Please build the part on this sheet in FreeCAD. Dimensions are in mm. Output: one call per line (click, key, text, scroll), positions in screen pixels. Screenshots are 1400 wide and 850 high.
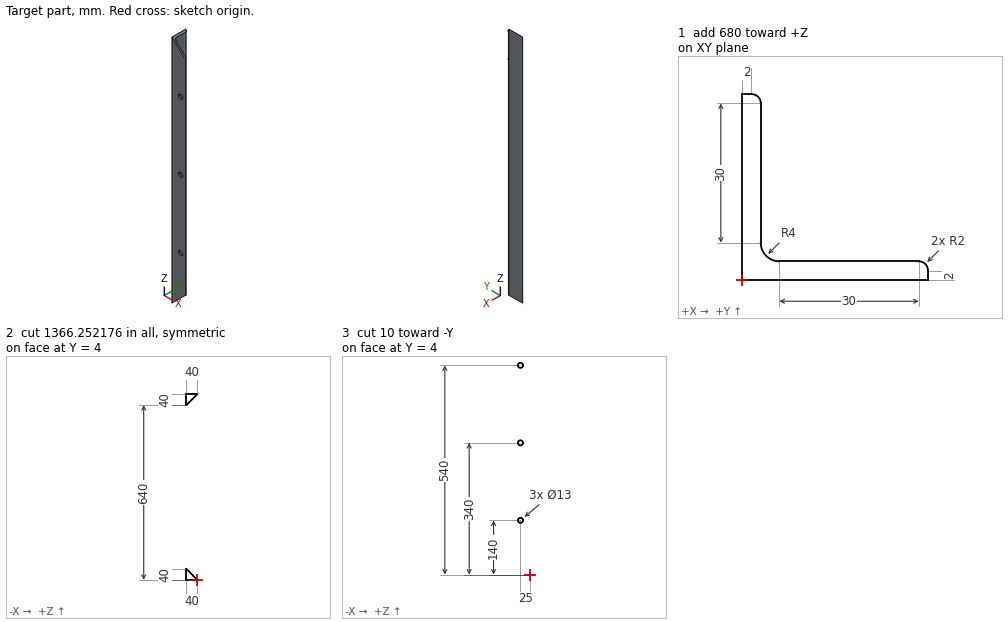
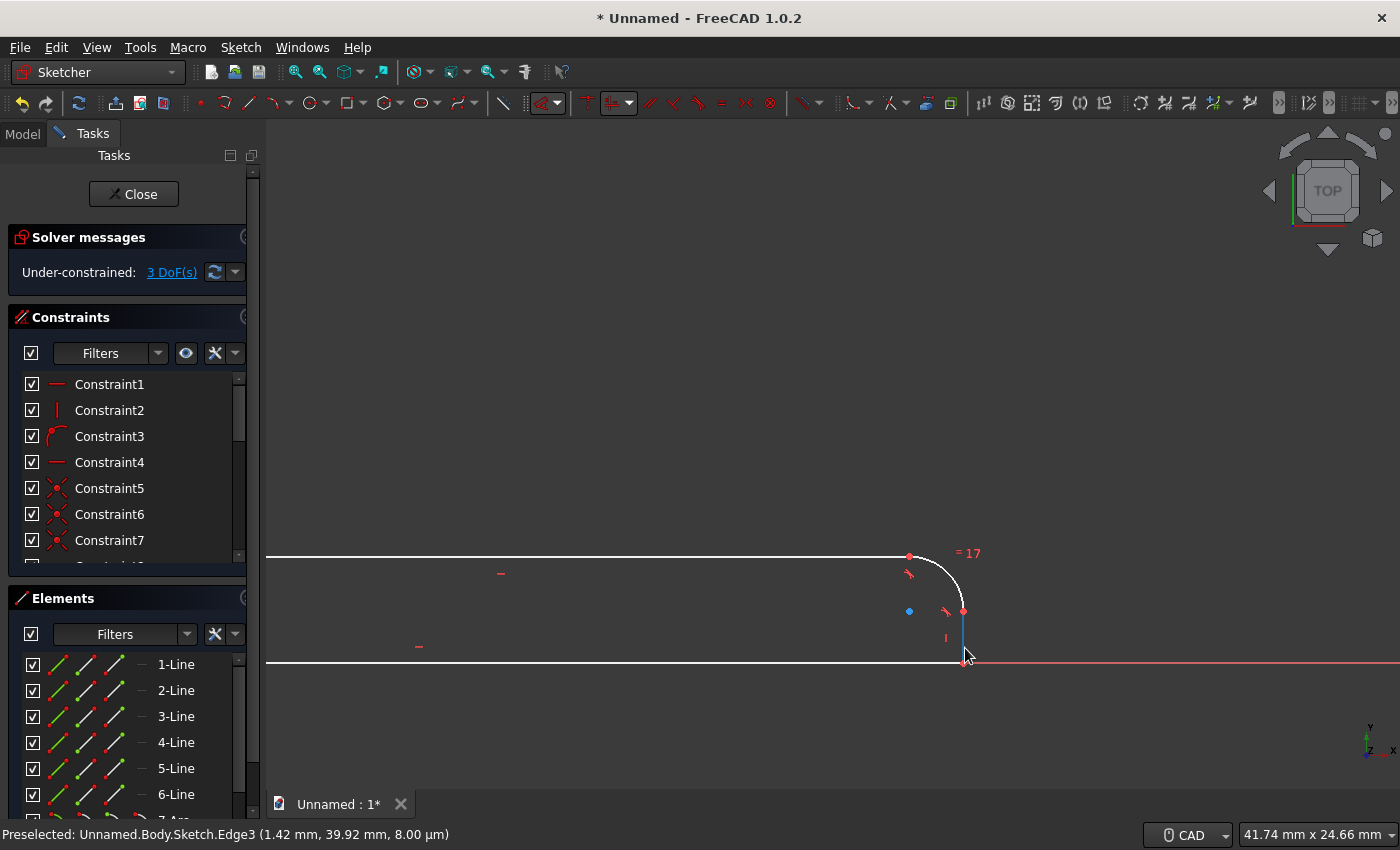
click(963, 648)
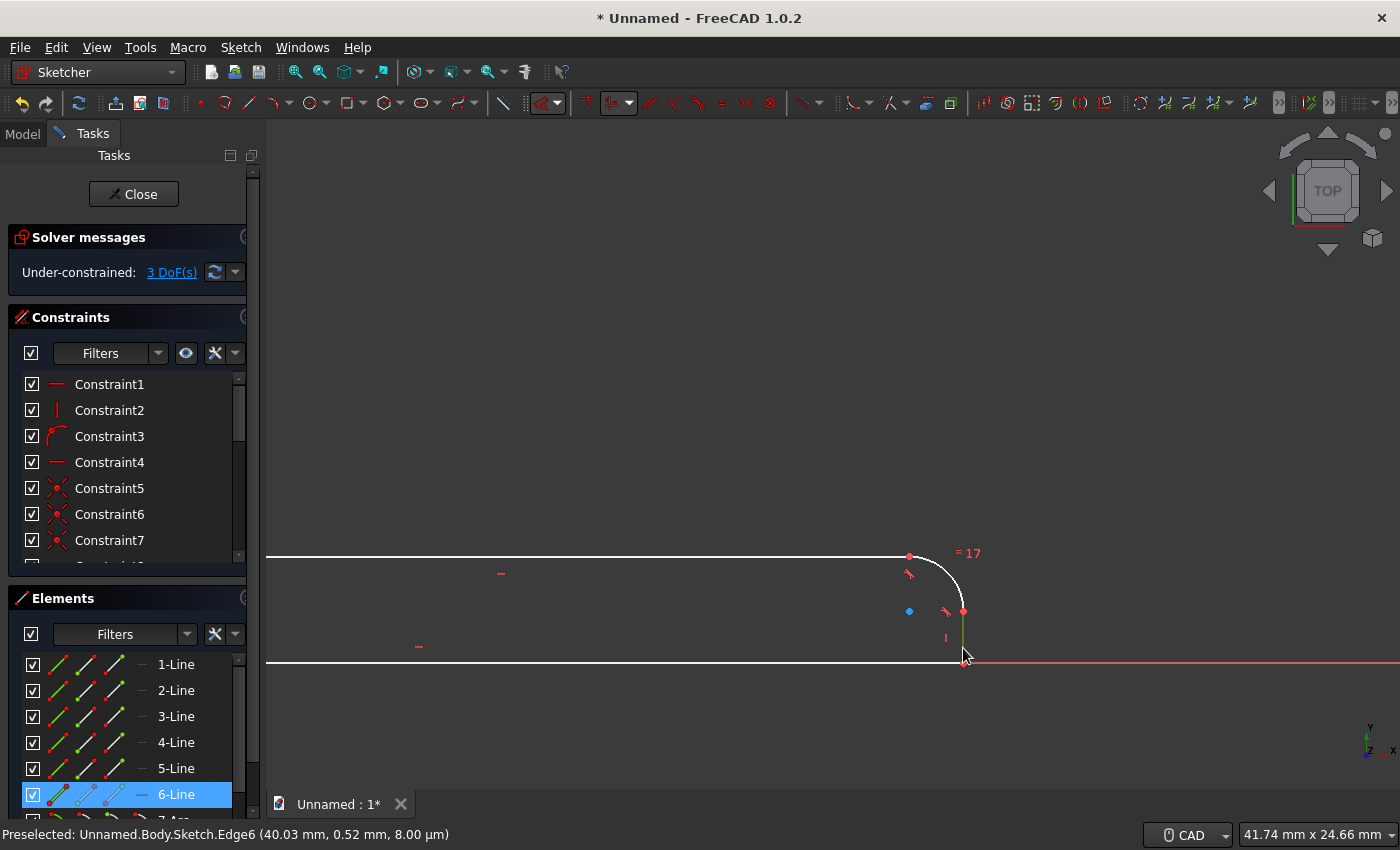
click(560, 104)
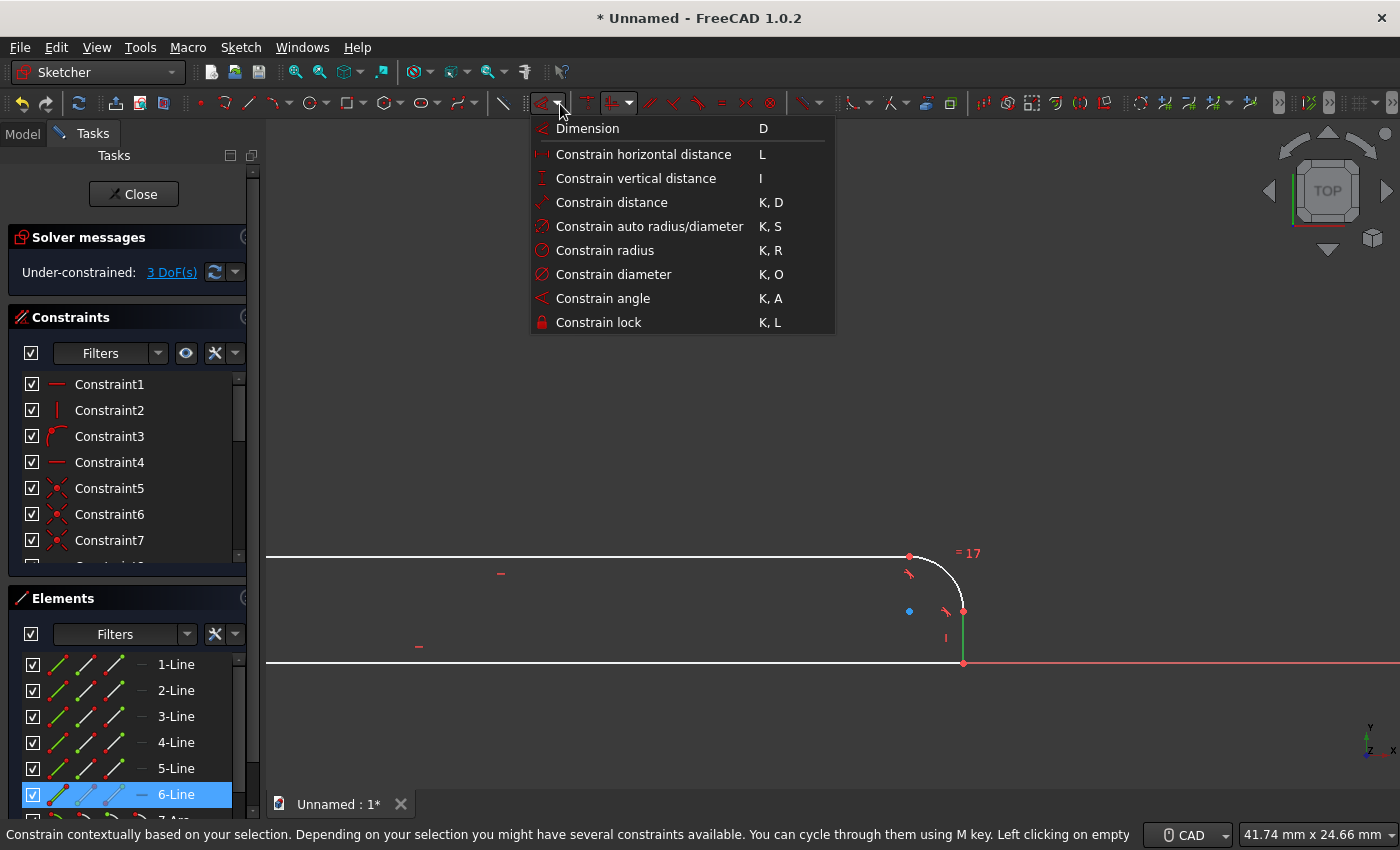
click(683, 178)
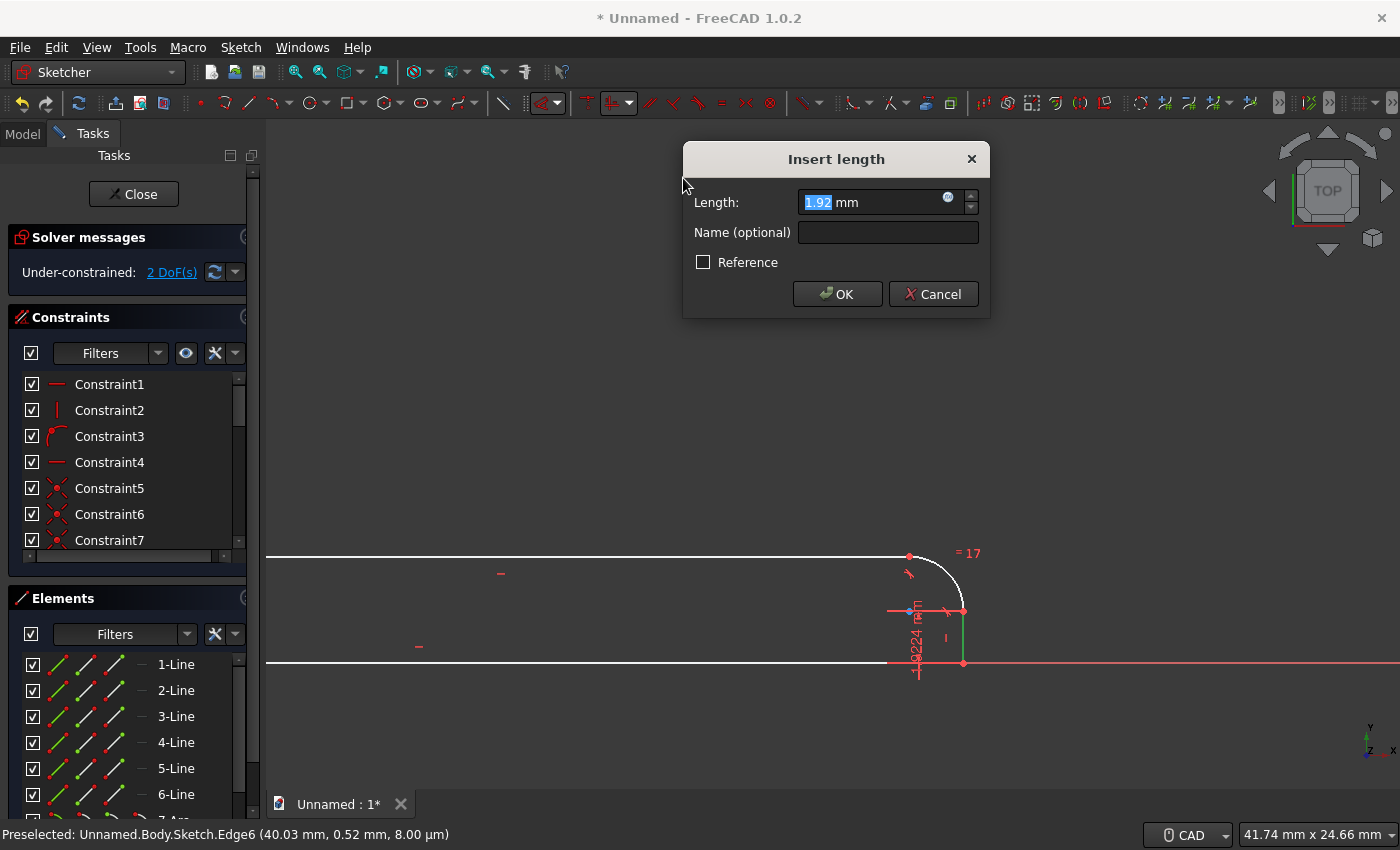
text(2)
key(Return)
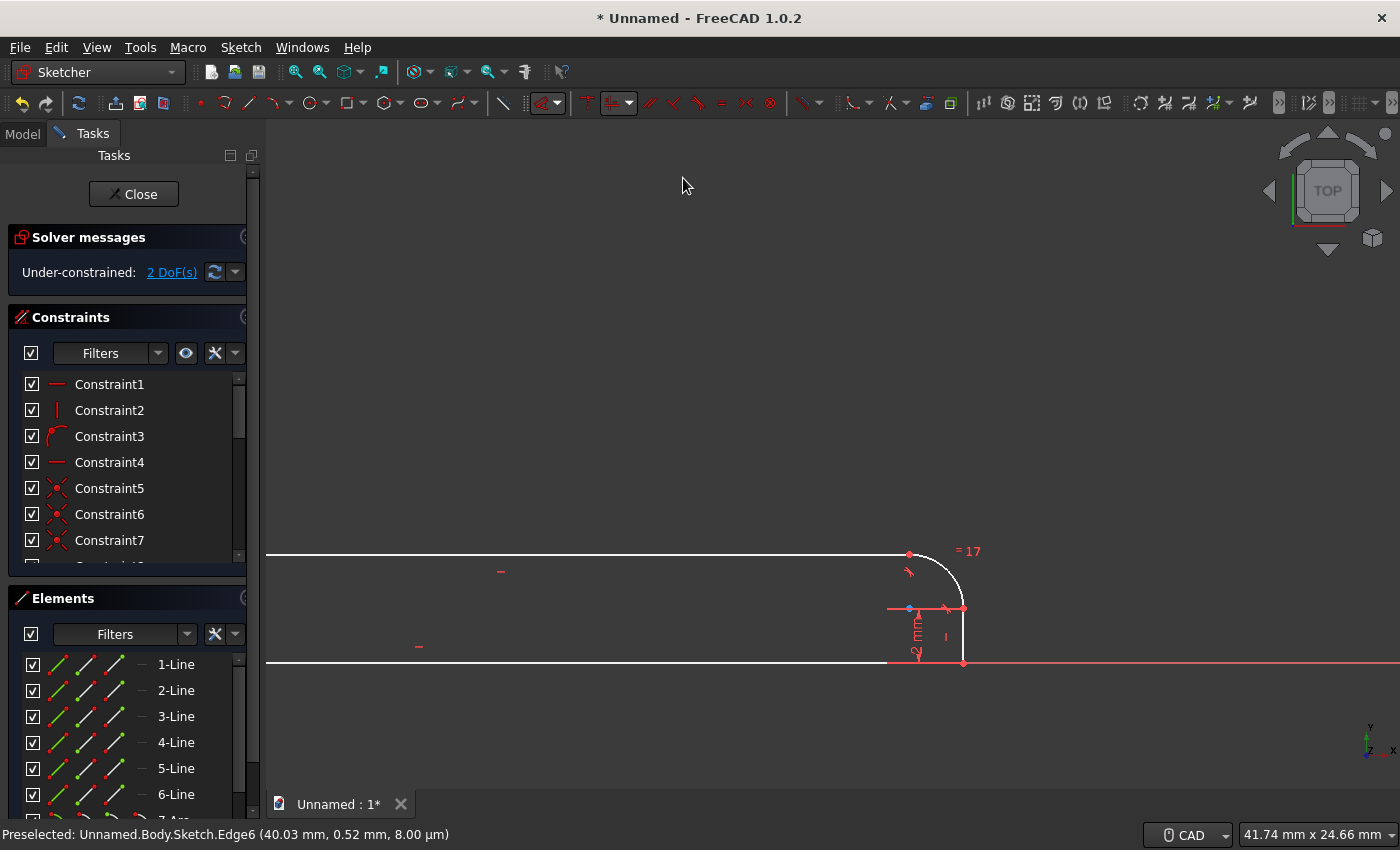
click(664, 555)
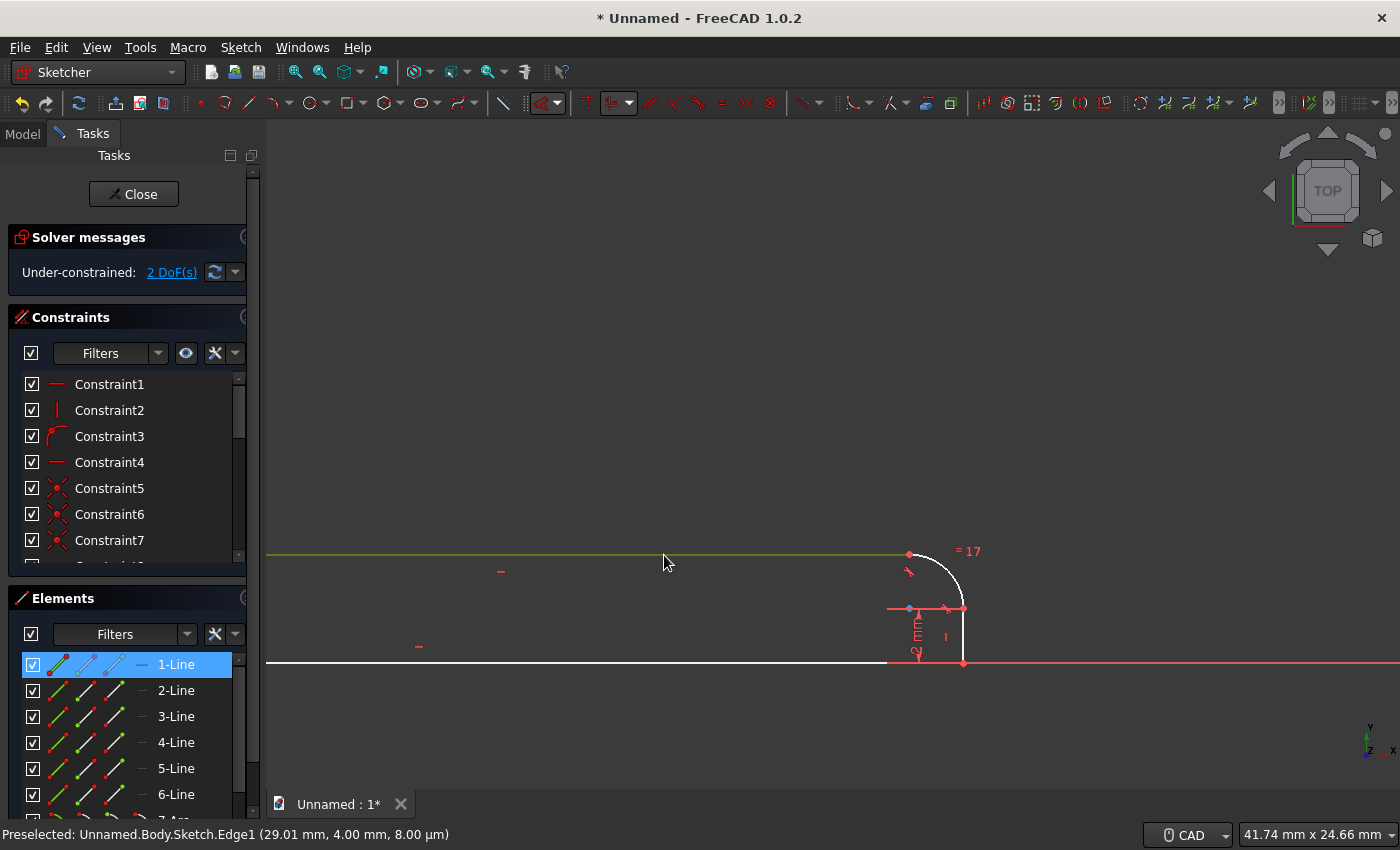
click(560, 104)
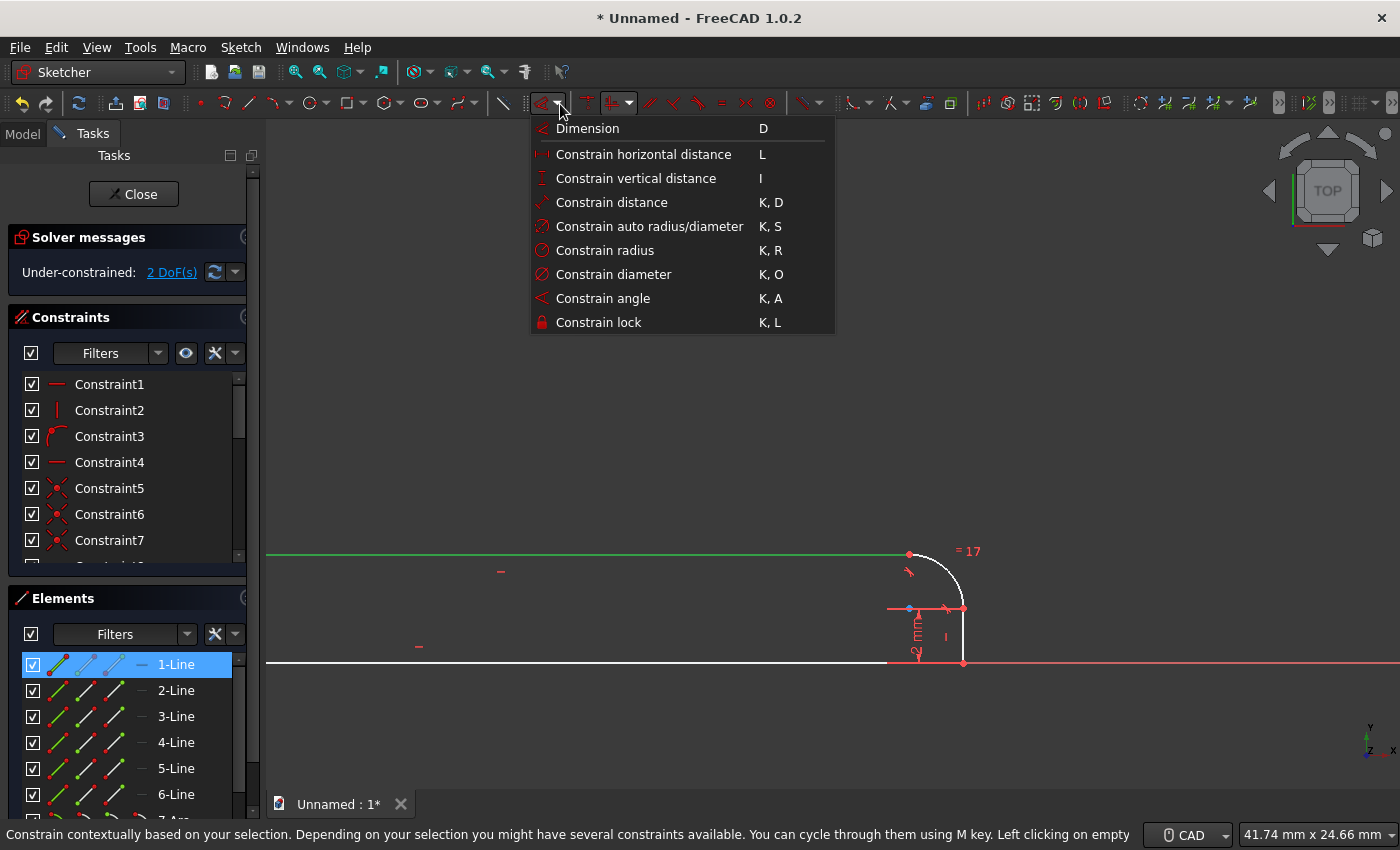
click(683, 154)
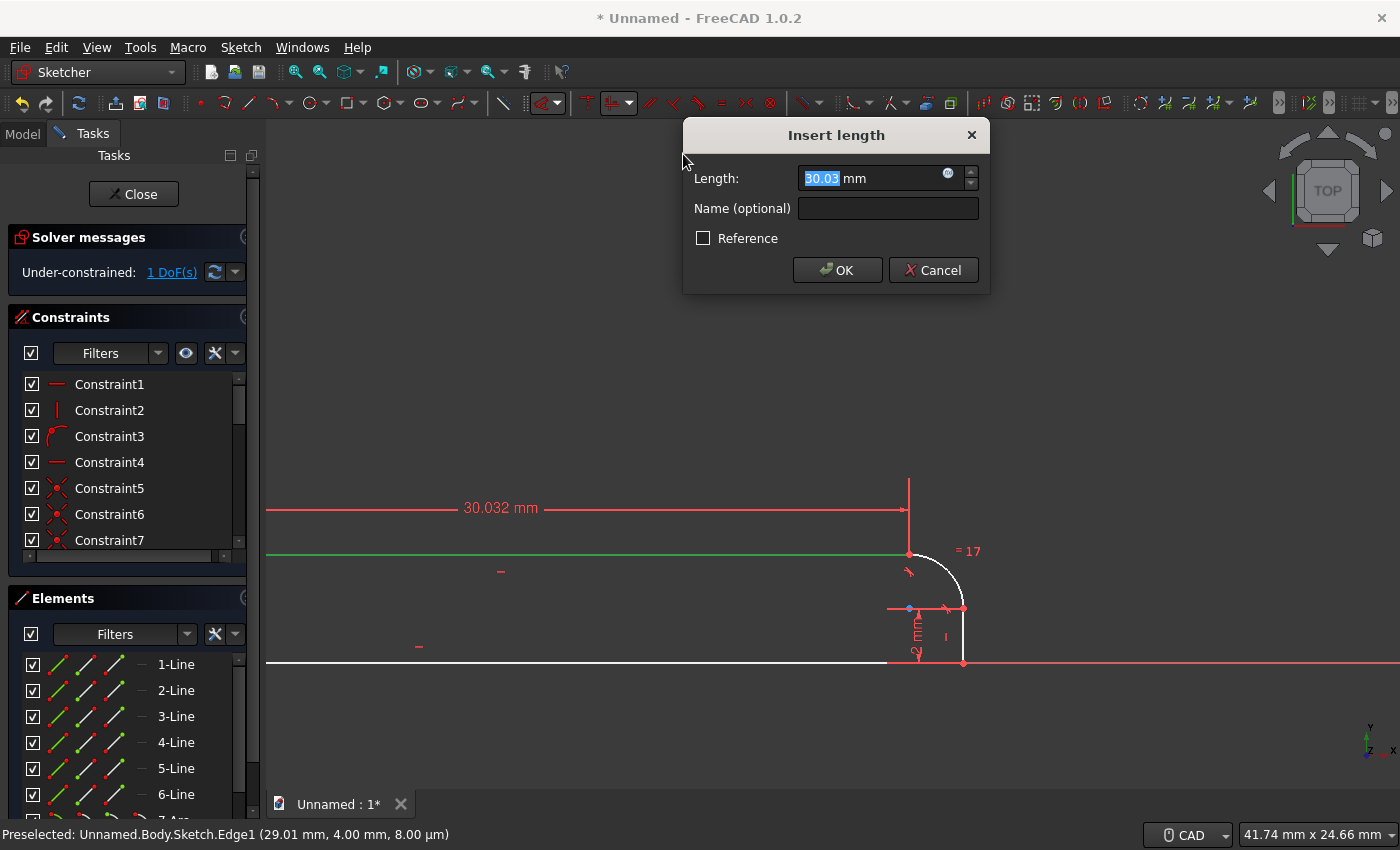
text(30)
key(Return)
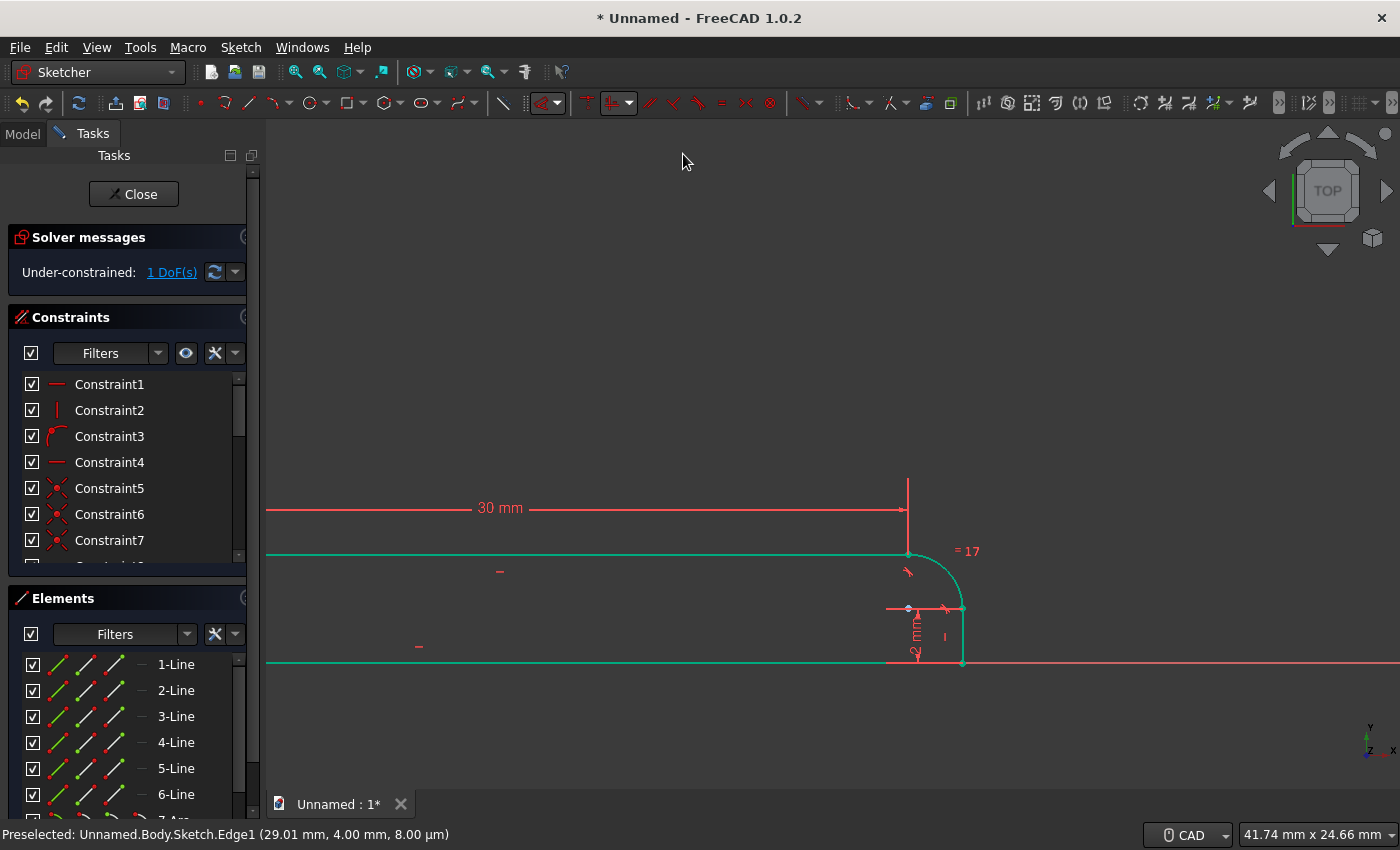
scroll(965, 648, down, 5)